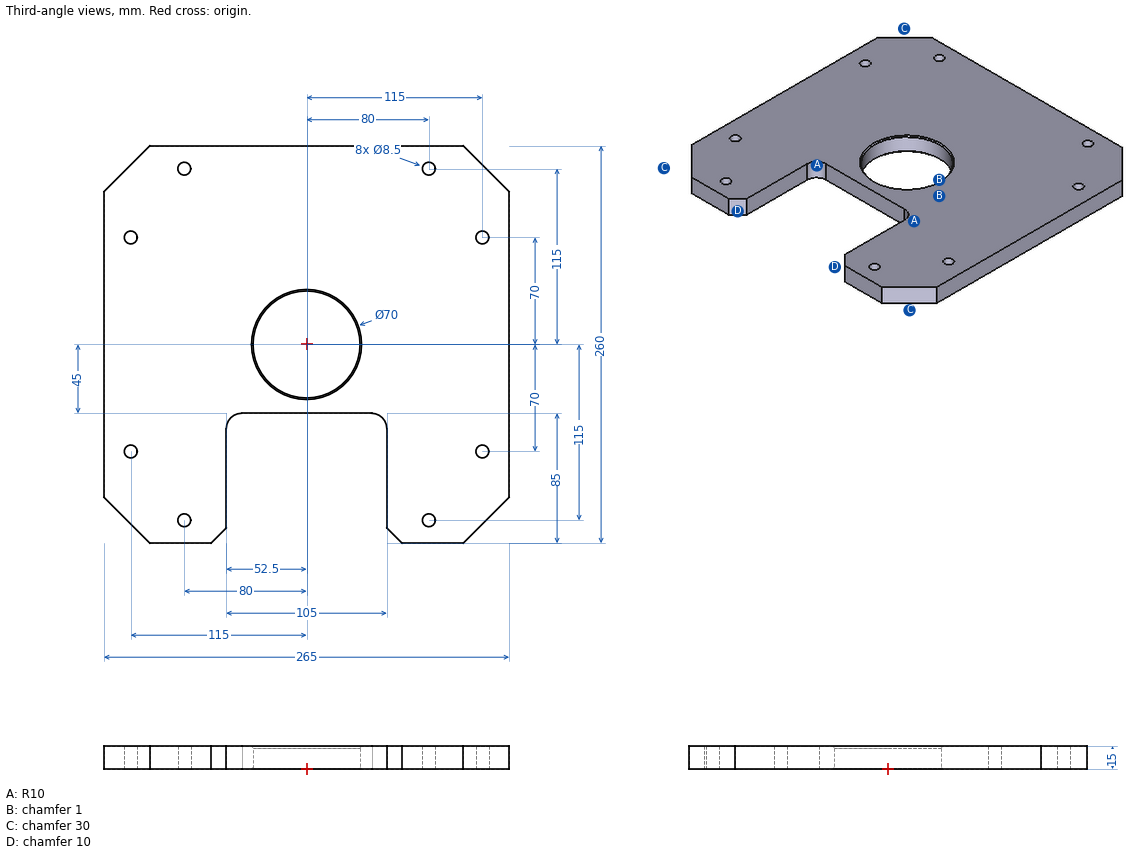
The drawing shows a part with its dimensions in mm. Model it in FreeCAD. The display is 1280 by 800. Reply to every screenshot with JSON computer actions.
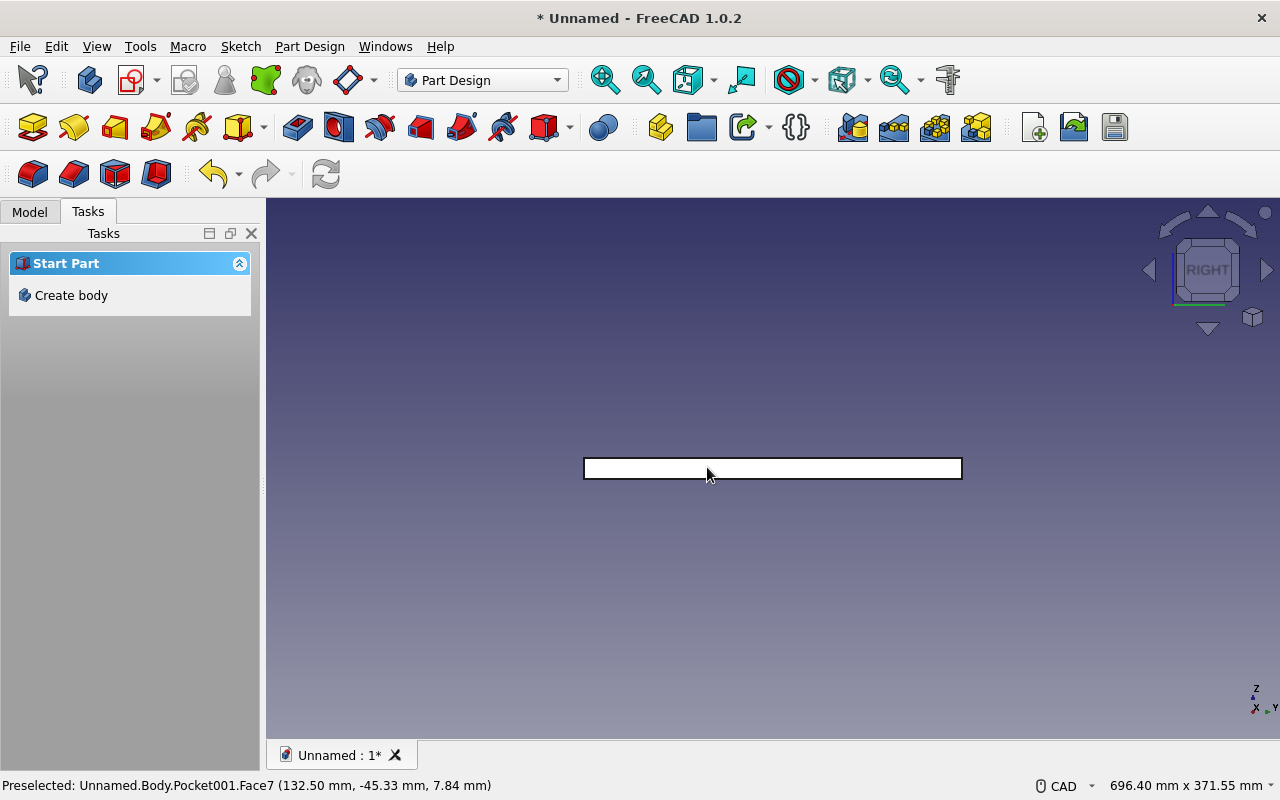
{"action": "key", "text": "5"}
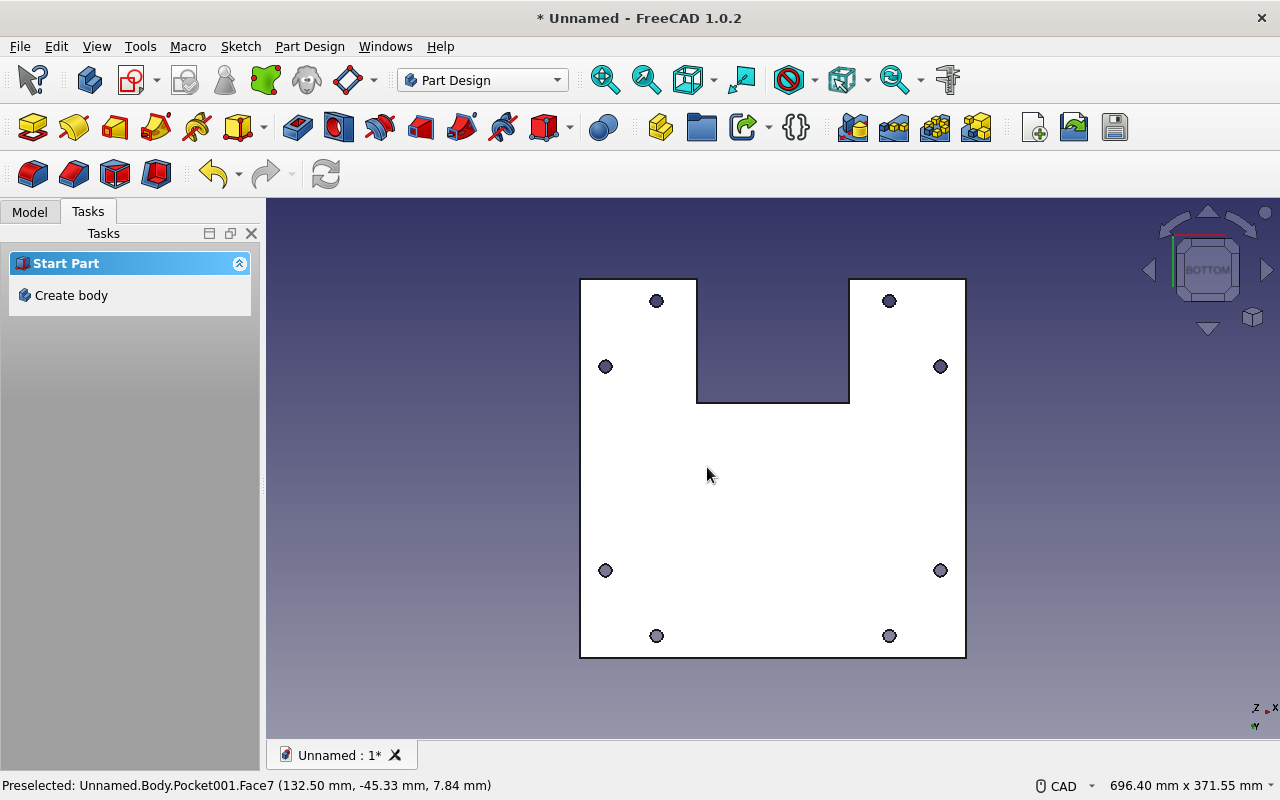
{"action": "scroll", "coordinate": [849, 402], "scroll_direction": "up", "scroll_amount": 4}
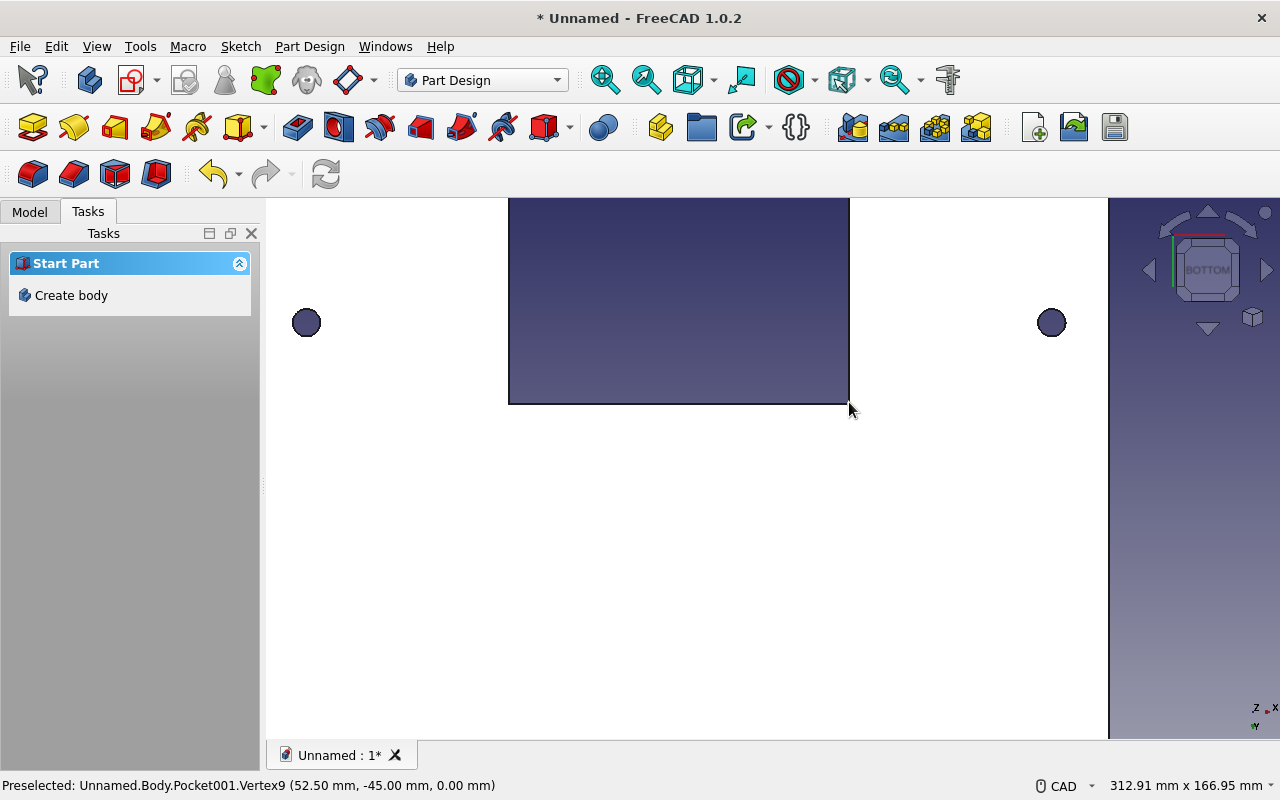
{"action": "left_click", "coordinate": [606, 80]}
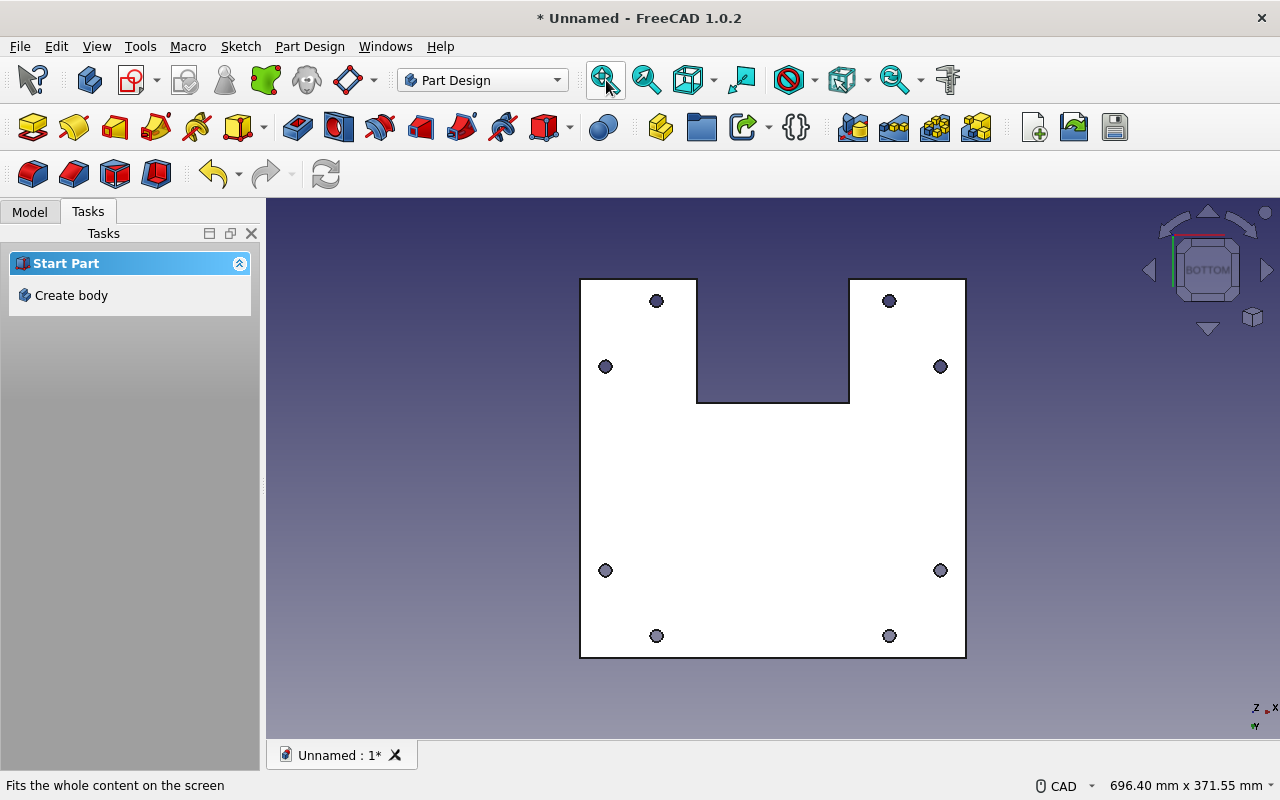
{"action": "key", "text": "4"}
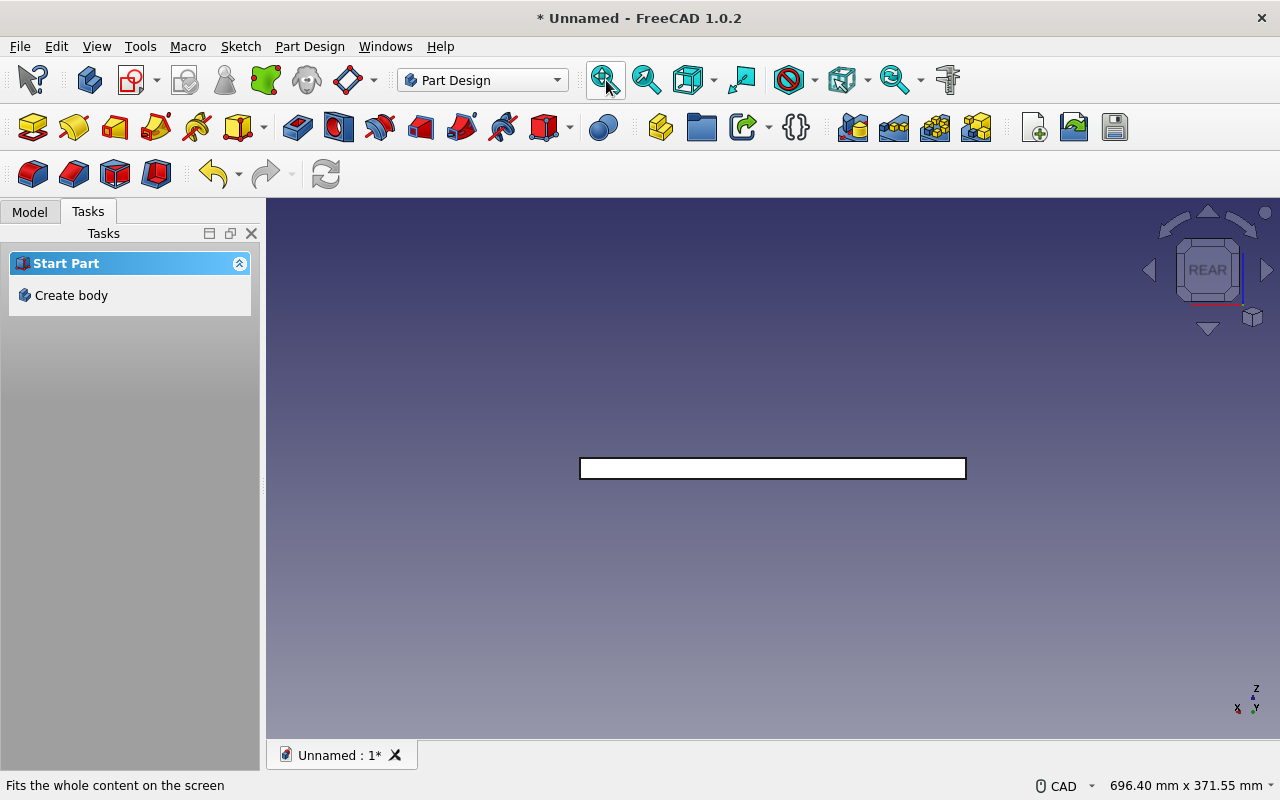
{"action": "left_click", "coordinate": [606, 80]}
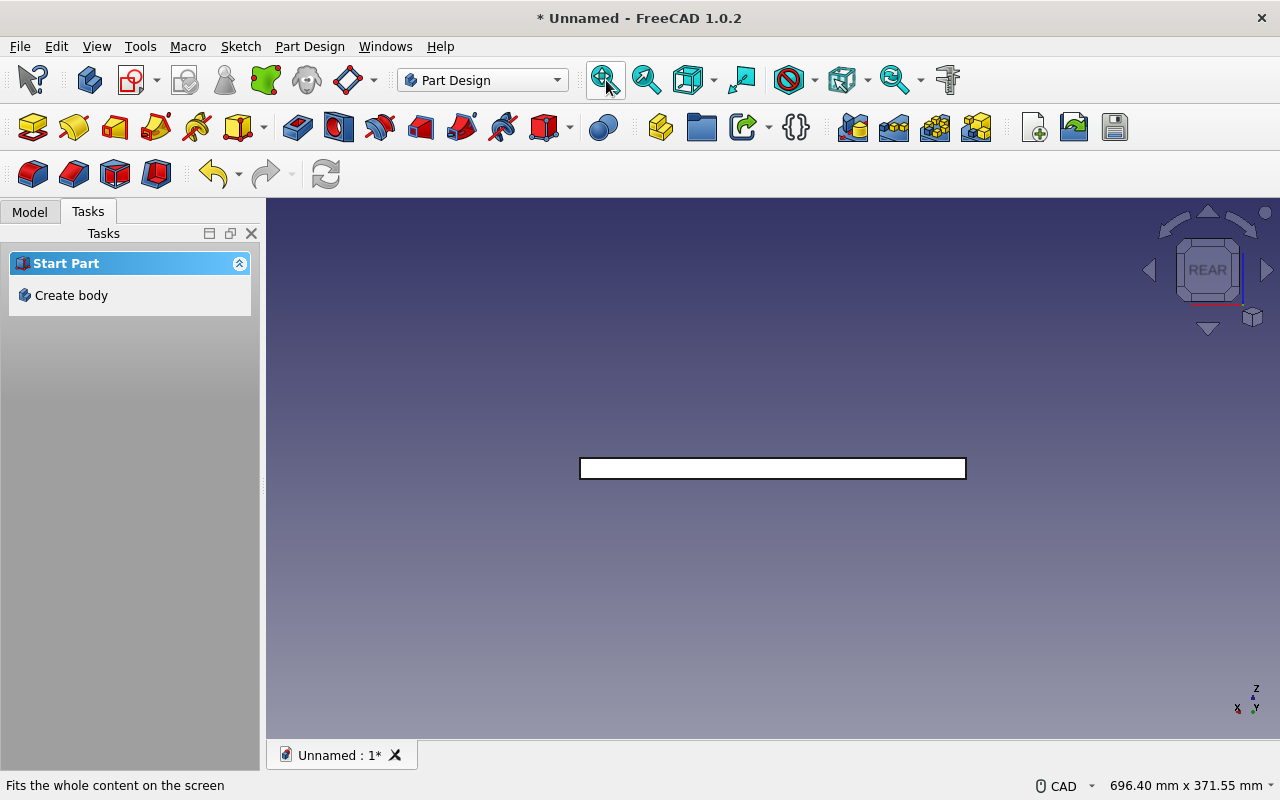
{"action": "scroll", "coordinate": [697, 468], "scroll_direction": "up", "scroll_amount": 4}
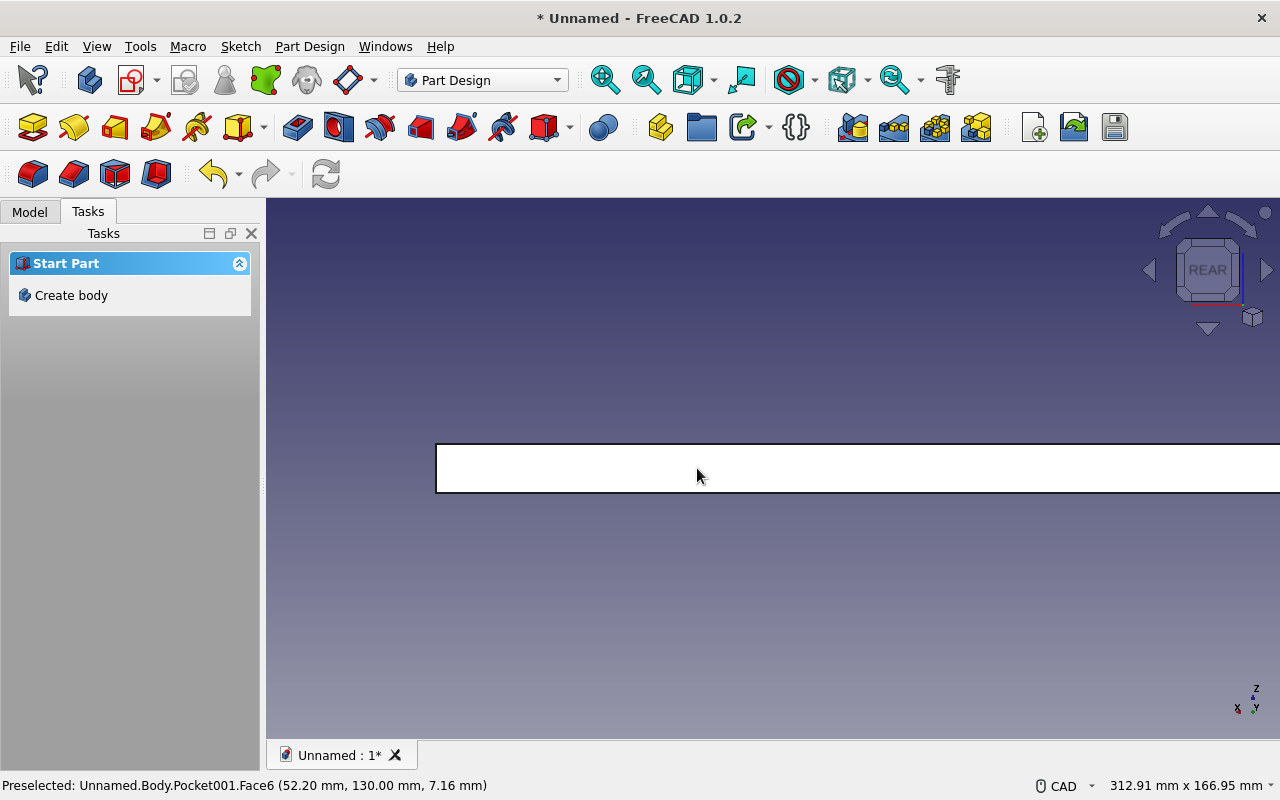
{"action": "left_click", "coordinate": [606, 80]}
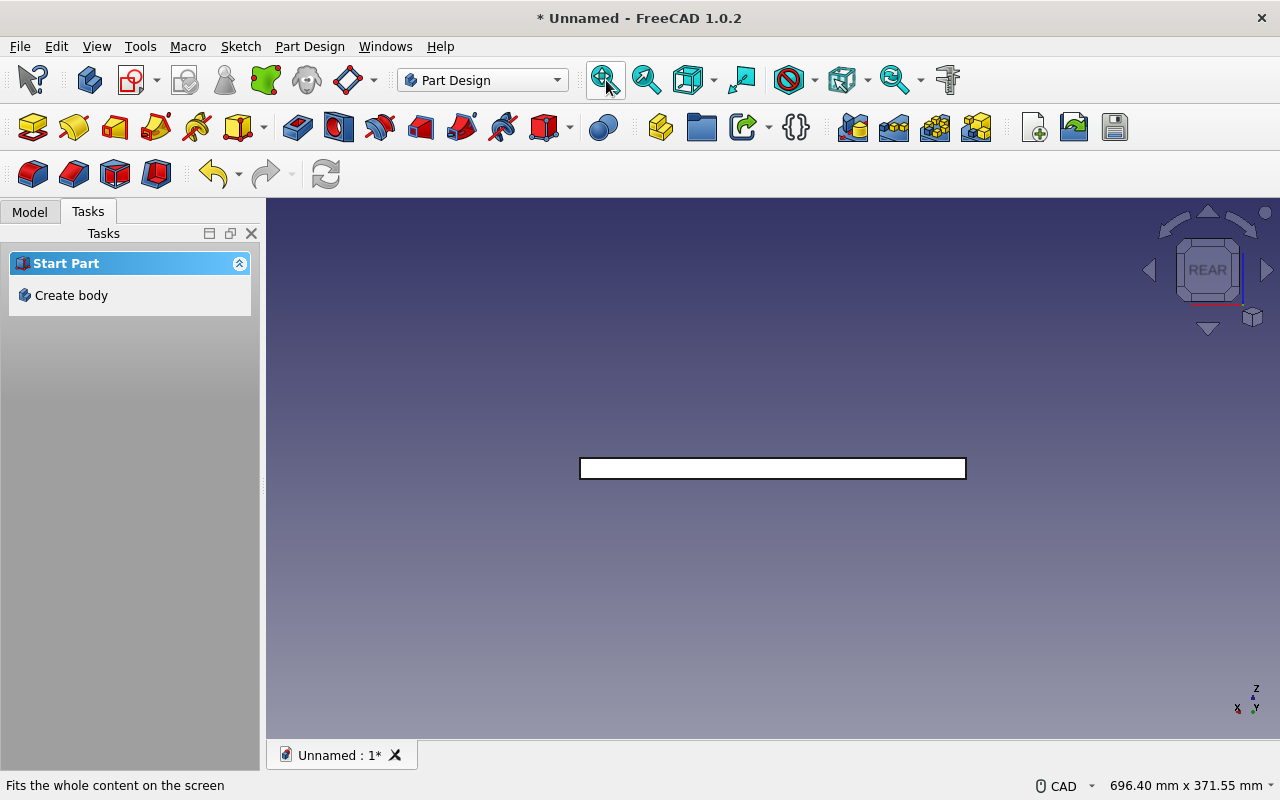
{"action": "key", "text": "6"}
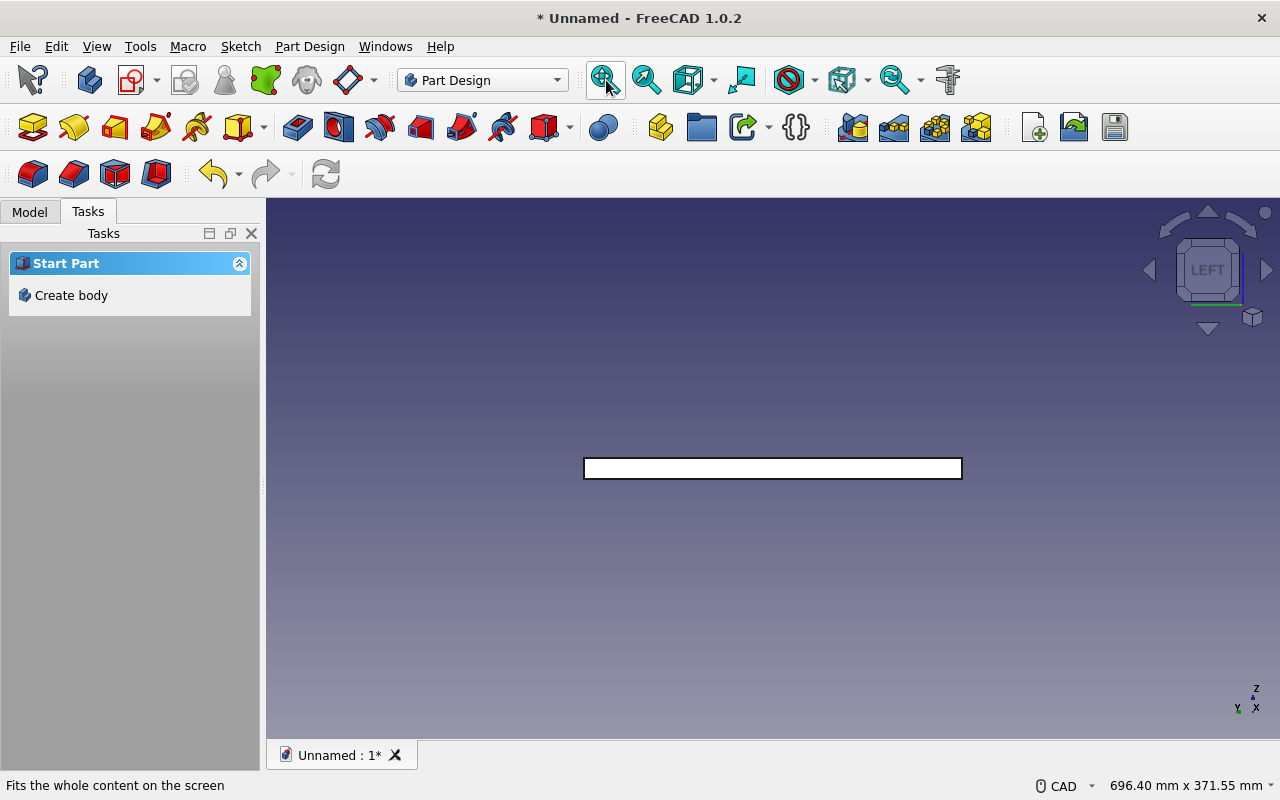
{"action": "left_click", "coordinate": [606, 80]}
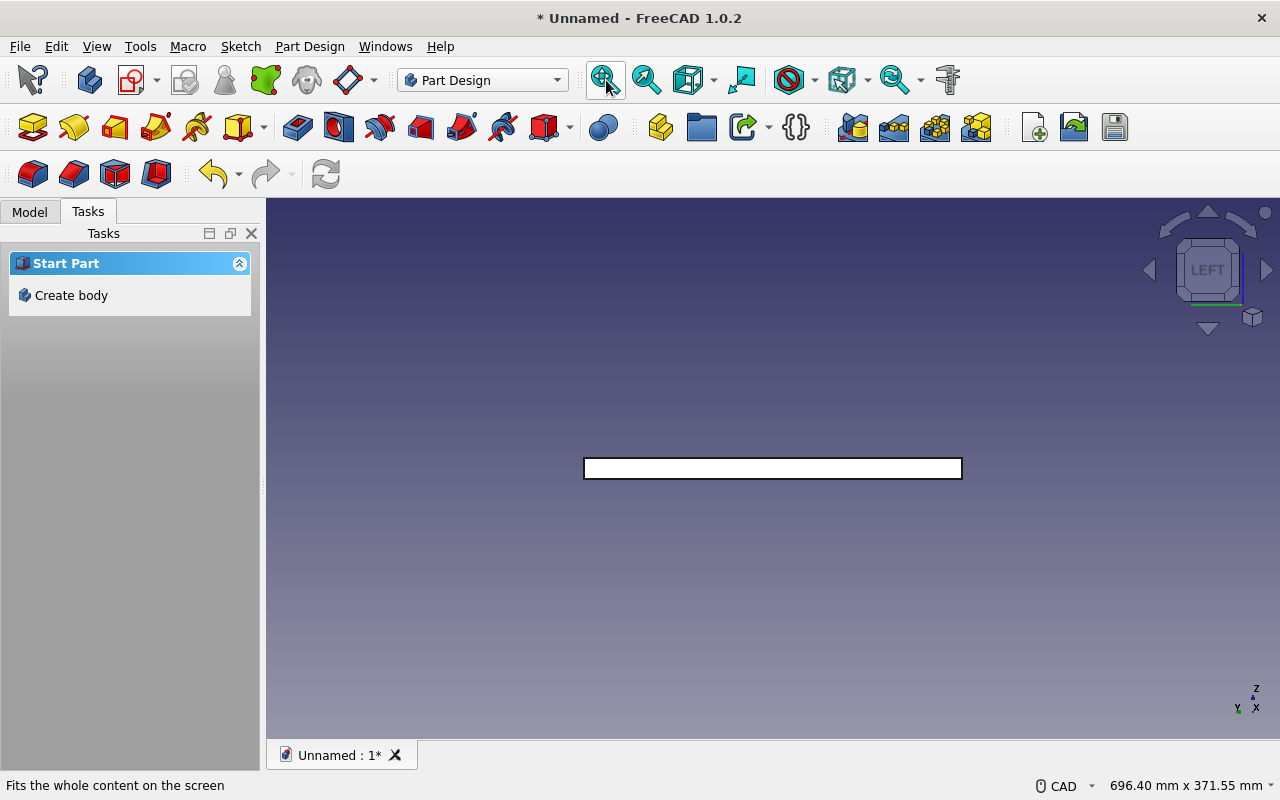
{"action": "scroll", "coordinate": [839, 467], "scroll_direction": "up", "scroll_amount": 4}